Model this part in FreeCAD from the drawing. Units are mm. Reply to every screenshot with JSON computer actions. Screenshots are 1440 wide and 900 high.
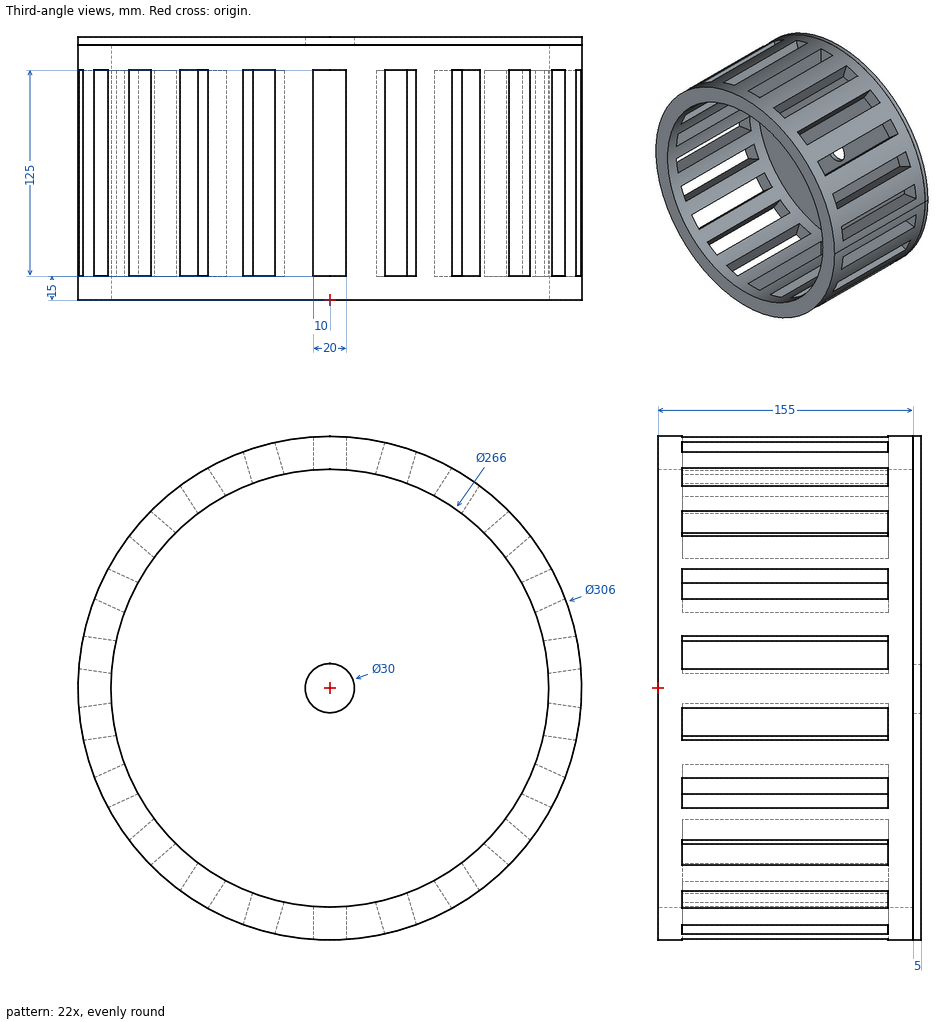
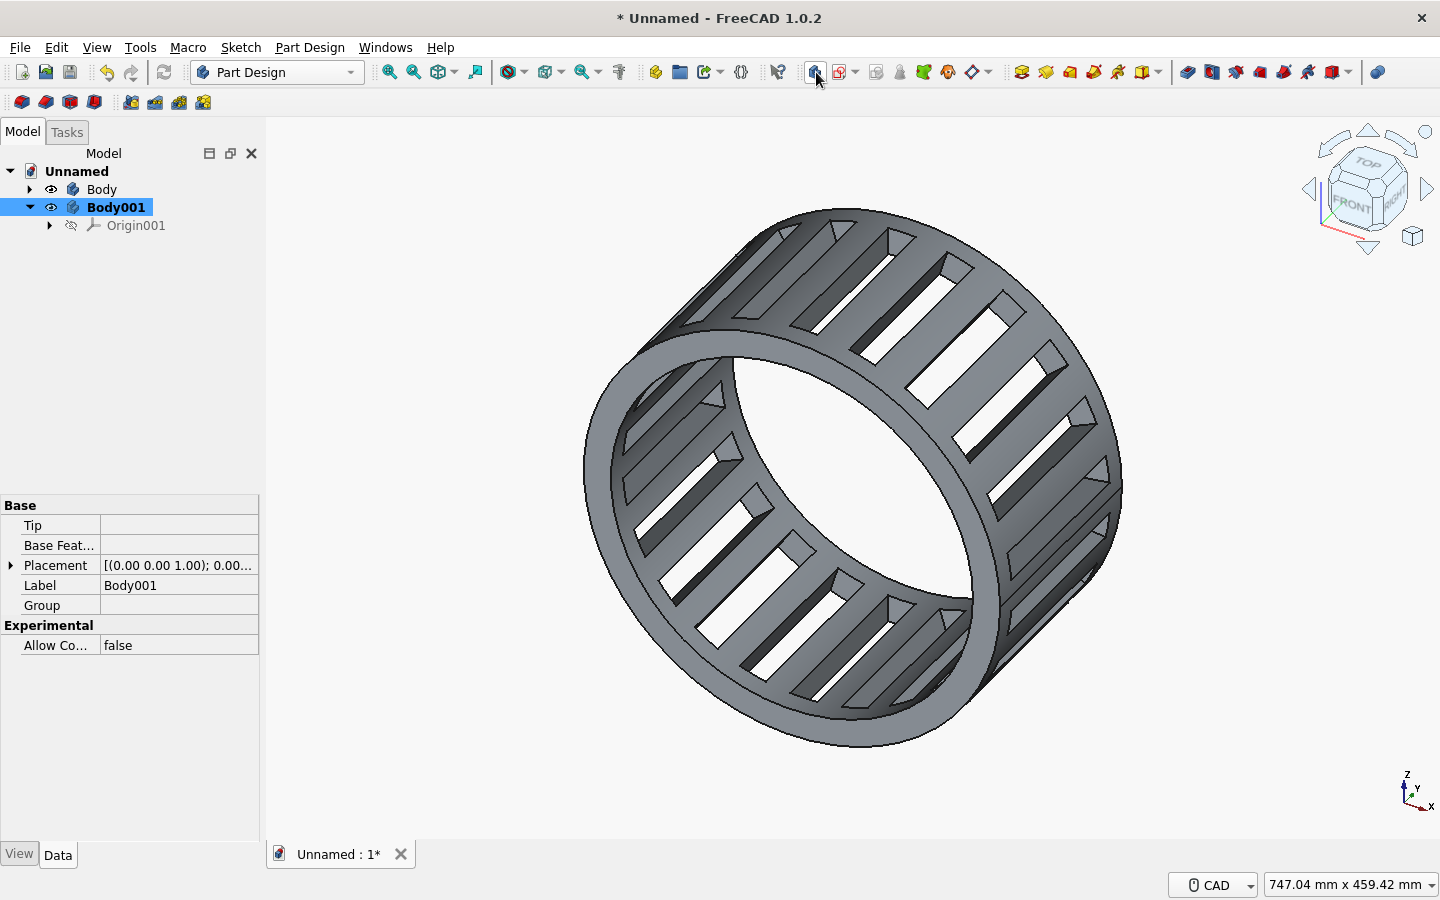
{"action": "left_click", "coordinate": [50, 225]}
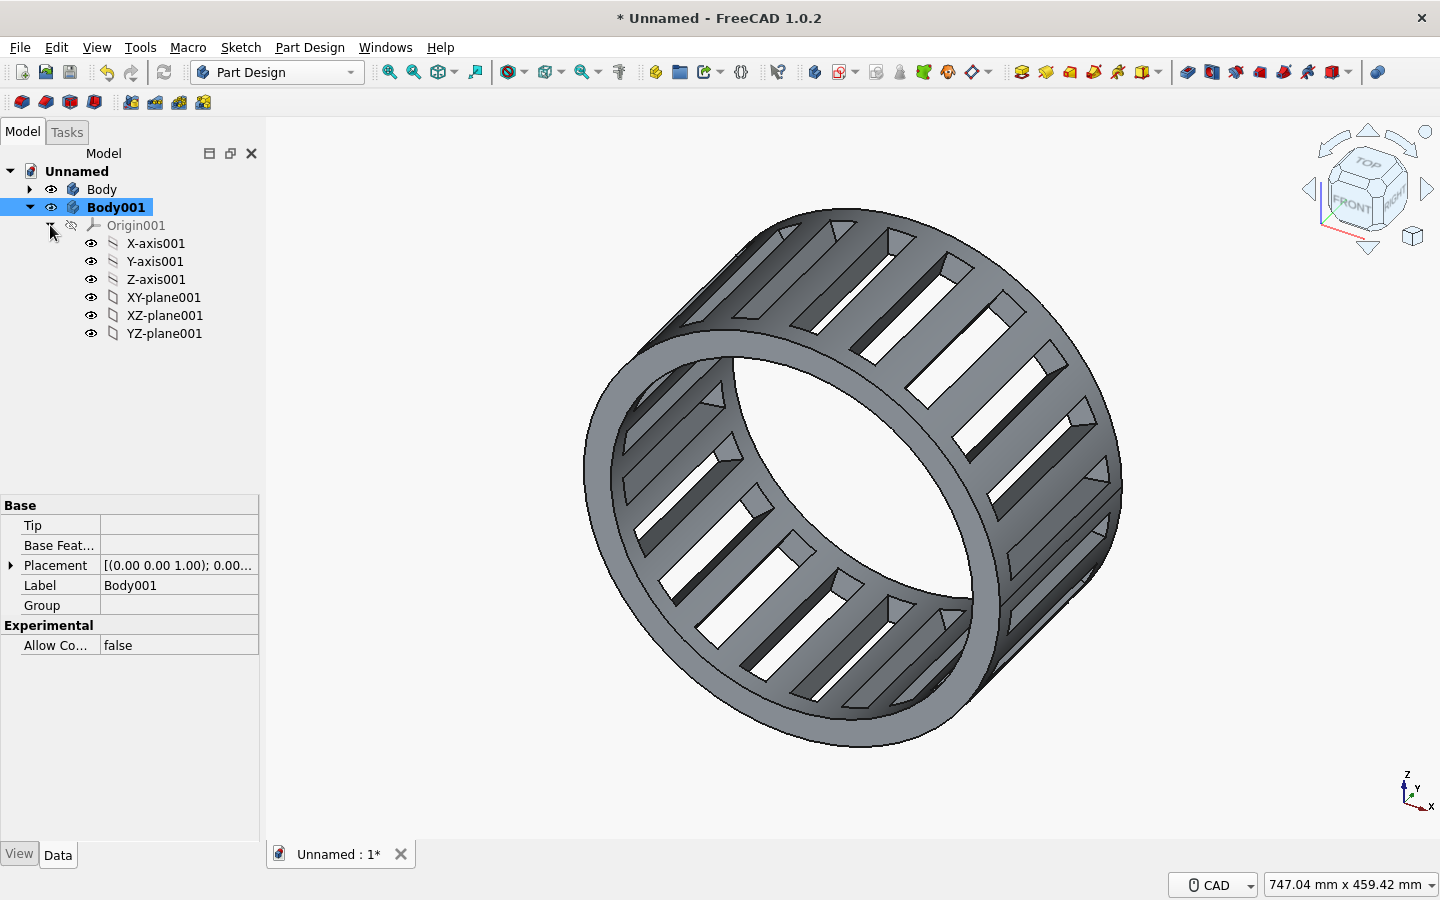
{"action": "left_click", "coordinate": [136, 315]}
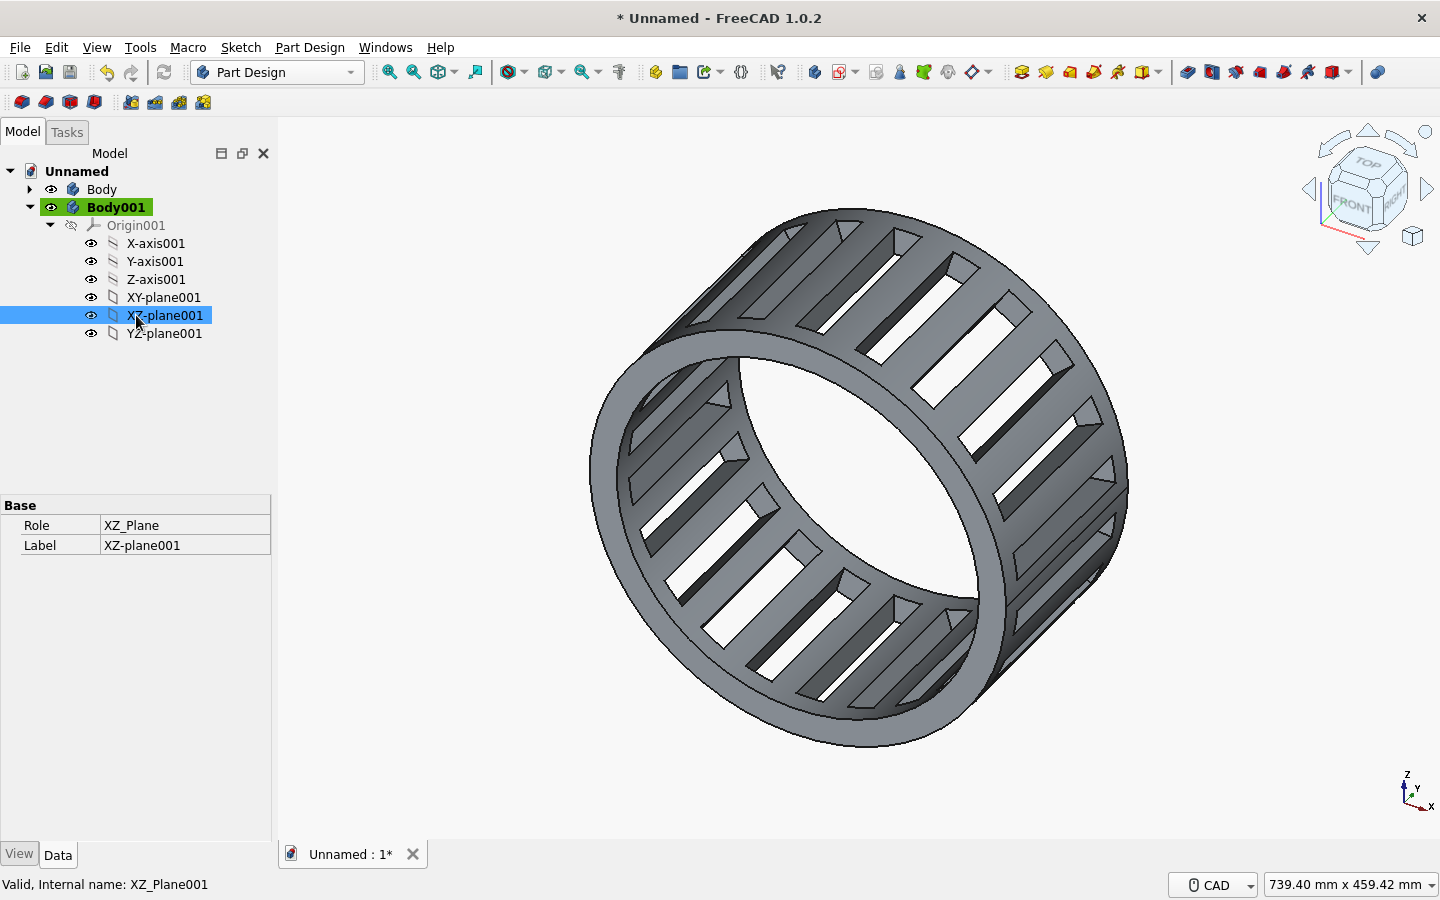
{"action": "left_click", "coordinate": [972, 72]}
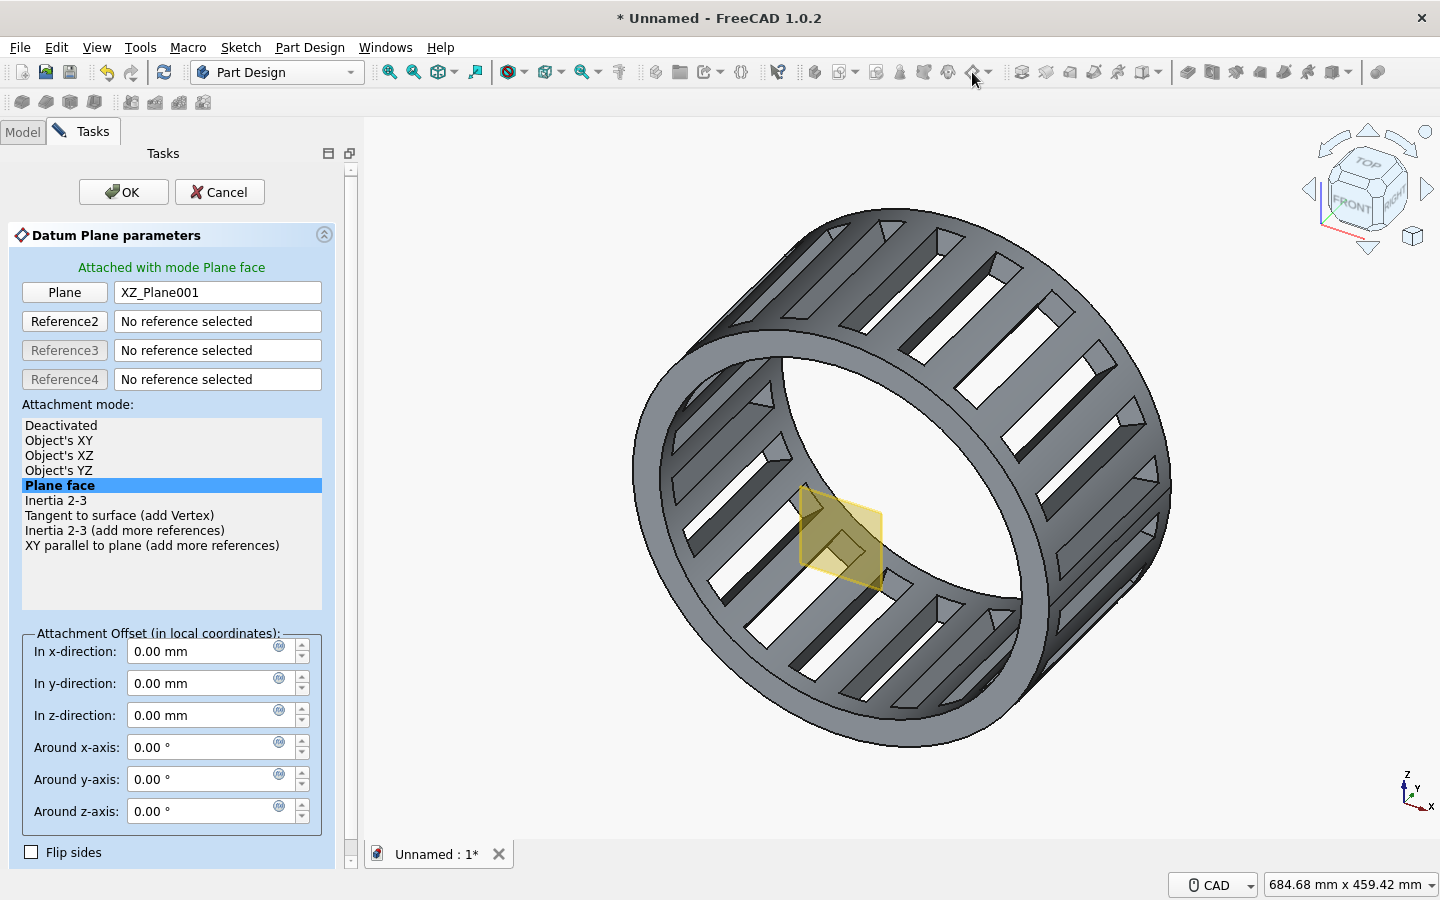
{"action": "triple_click", "coordinate": [210, 715]}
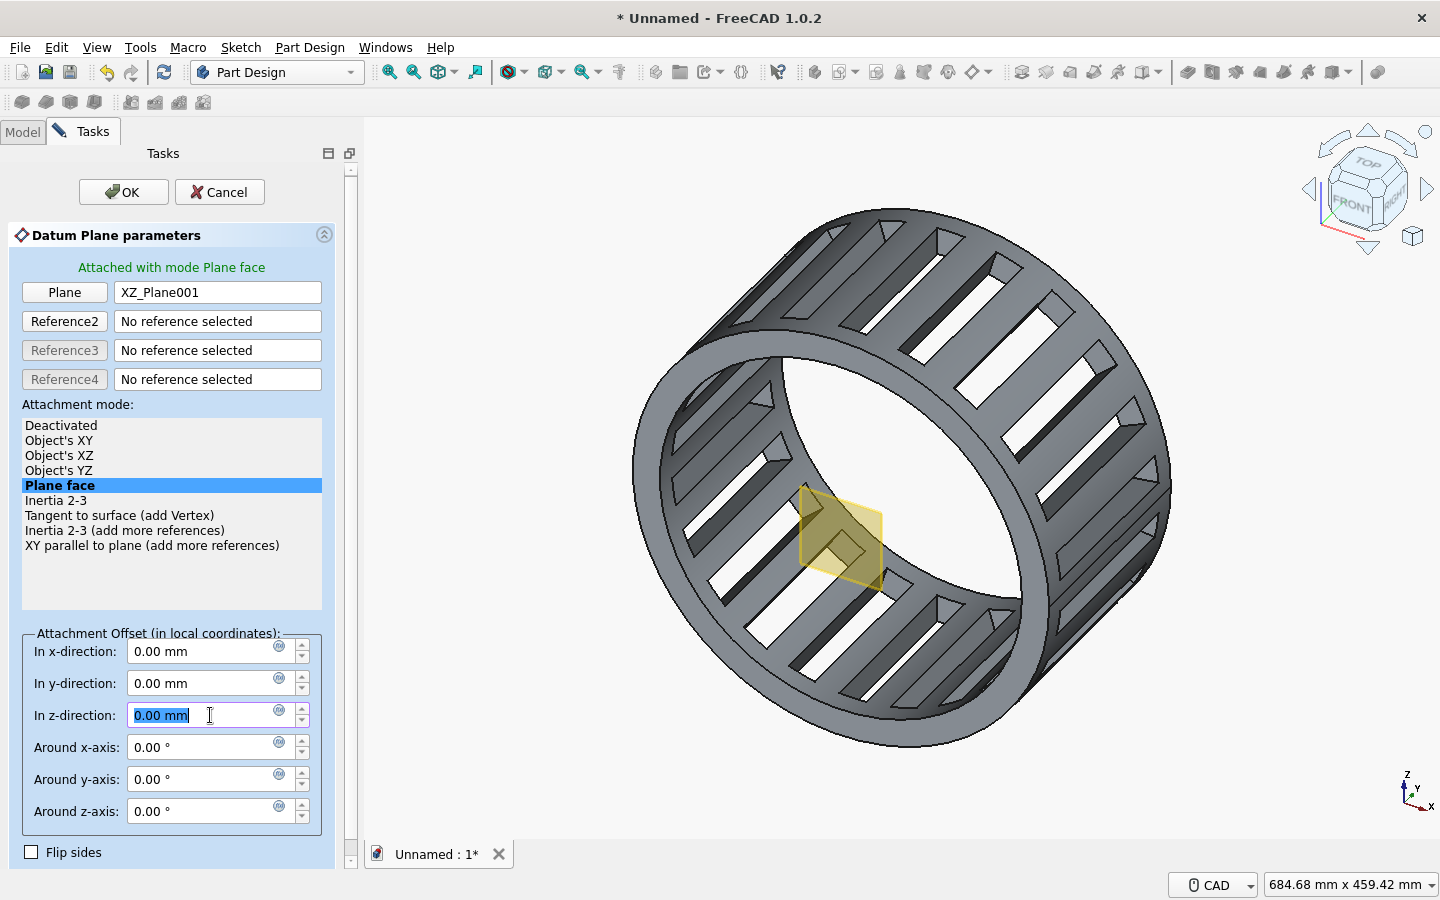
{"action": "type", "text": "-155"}
{"action": "key", "text": "Tab"}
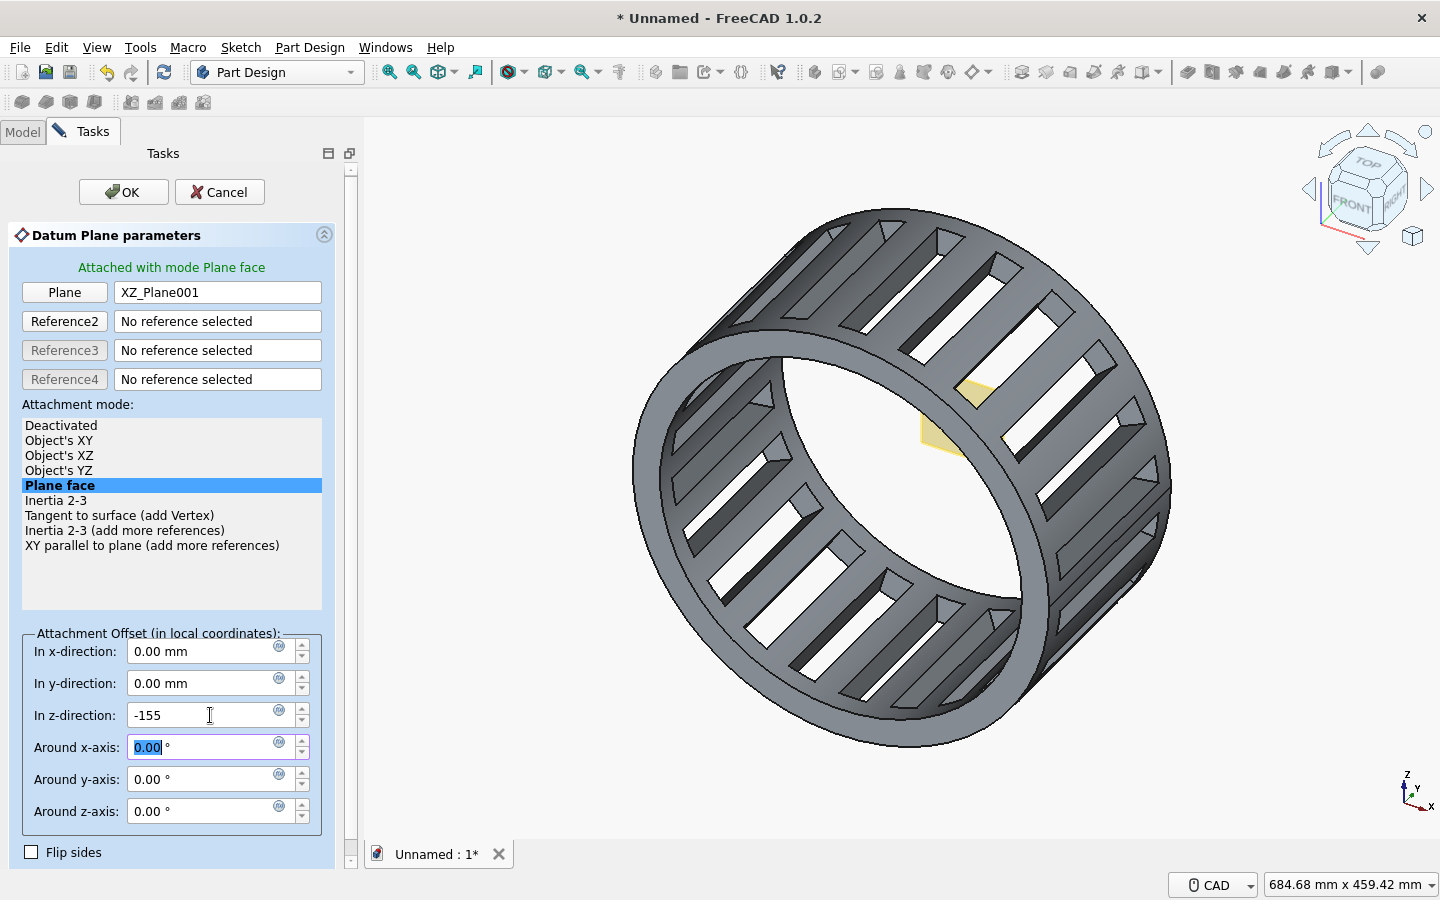
{"action": "left_click", "coordinate": [124, 192]}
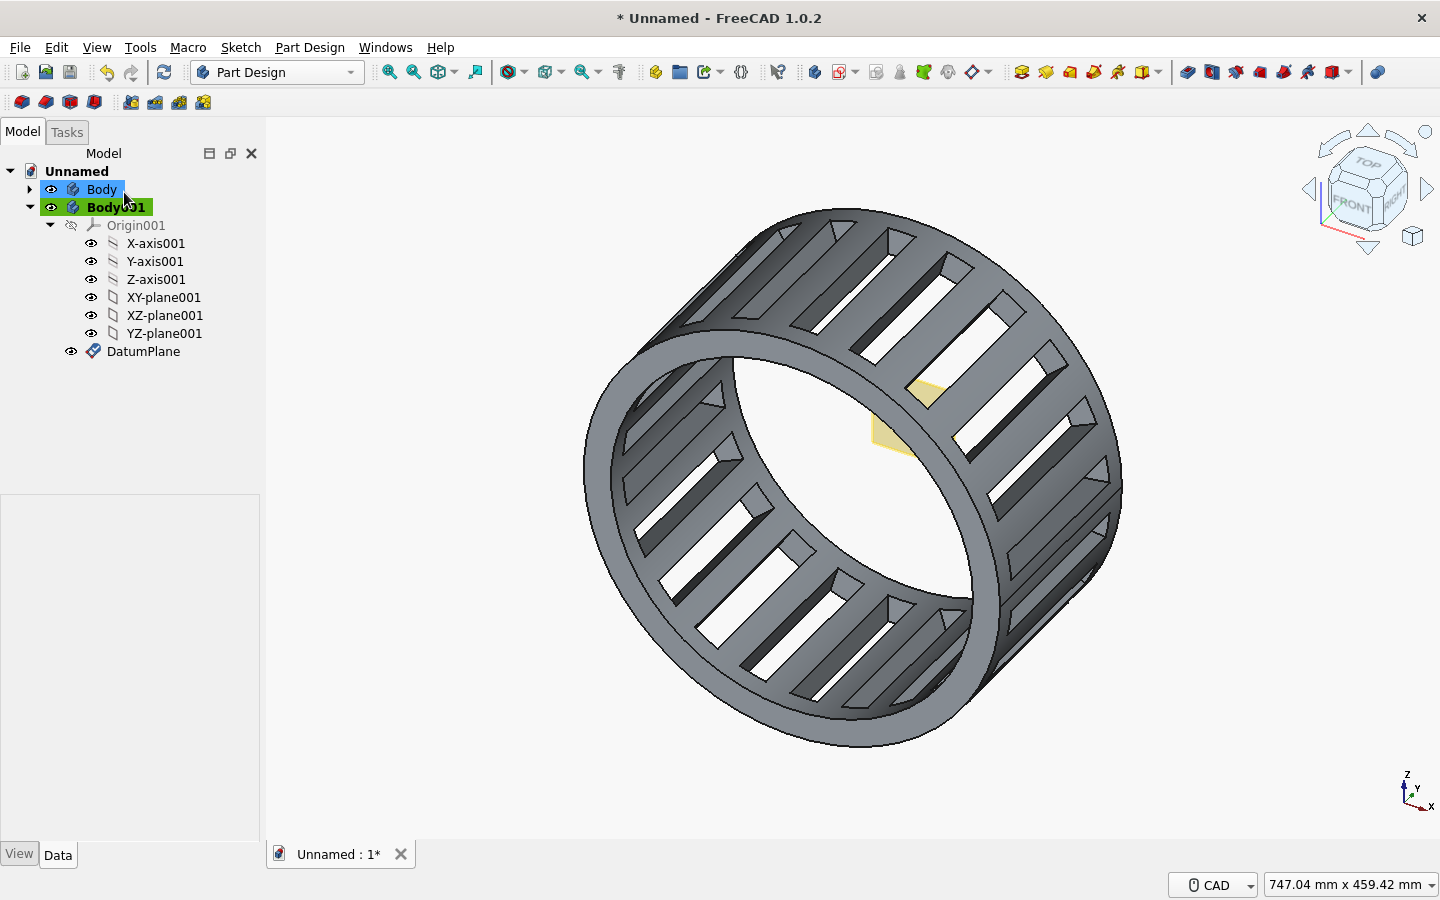
{"action": "left_click", "coordinate": [116, 351]}